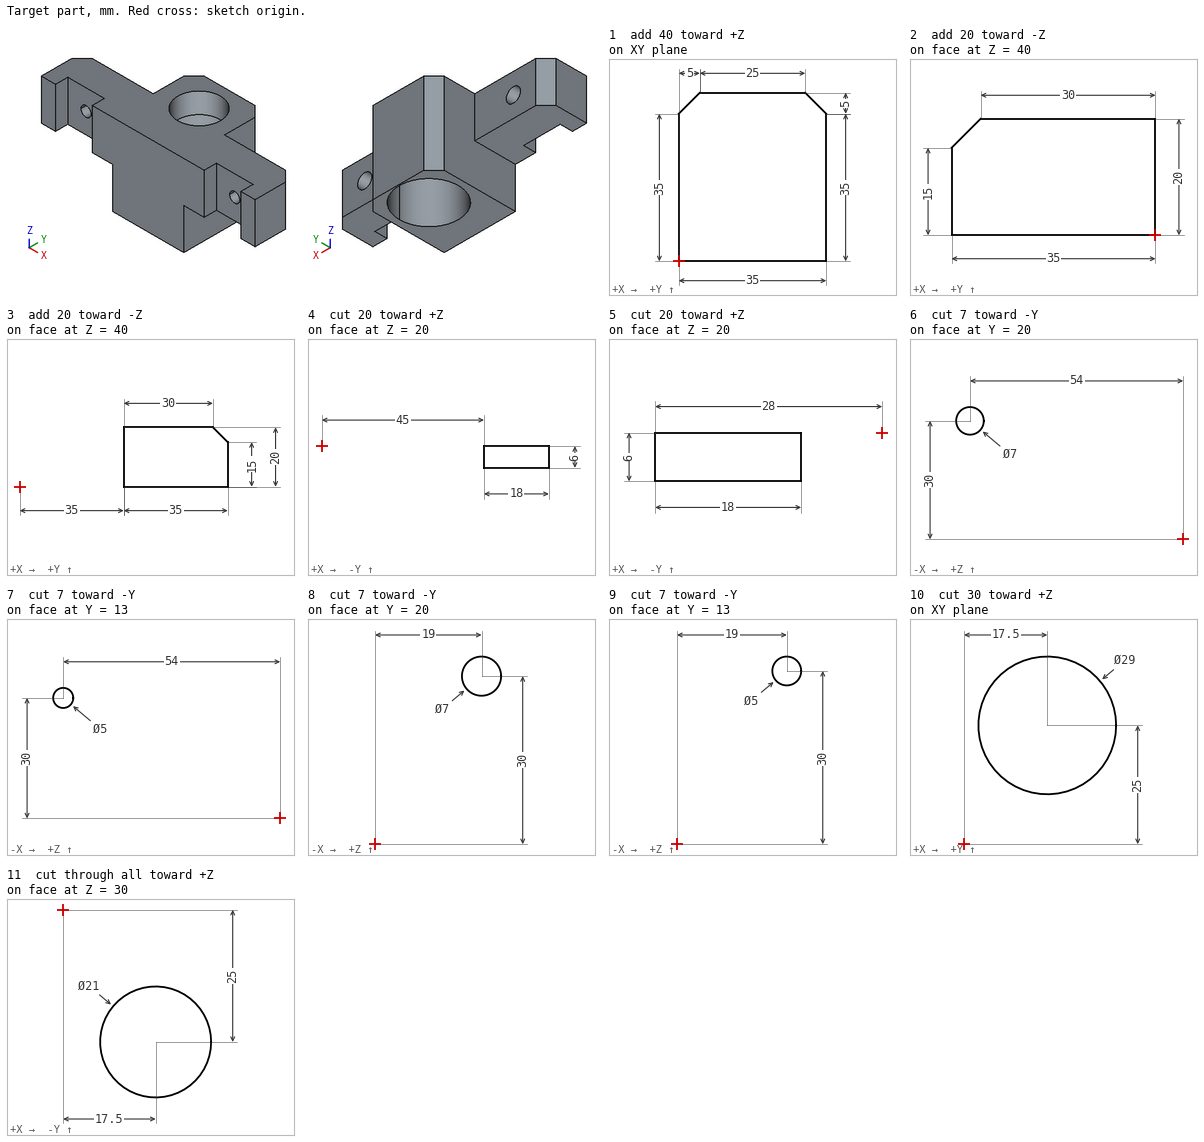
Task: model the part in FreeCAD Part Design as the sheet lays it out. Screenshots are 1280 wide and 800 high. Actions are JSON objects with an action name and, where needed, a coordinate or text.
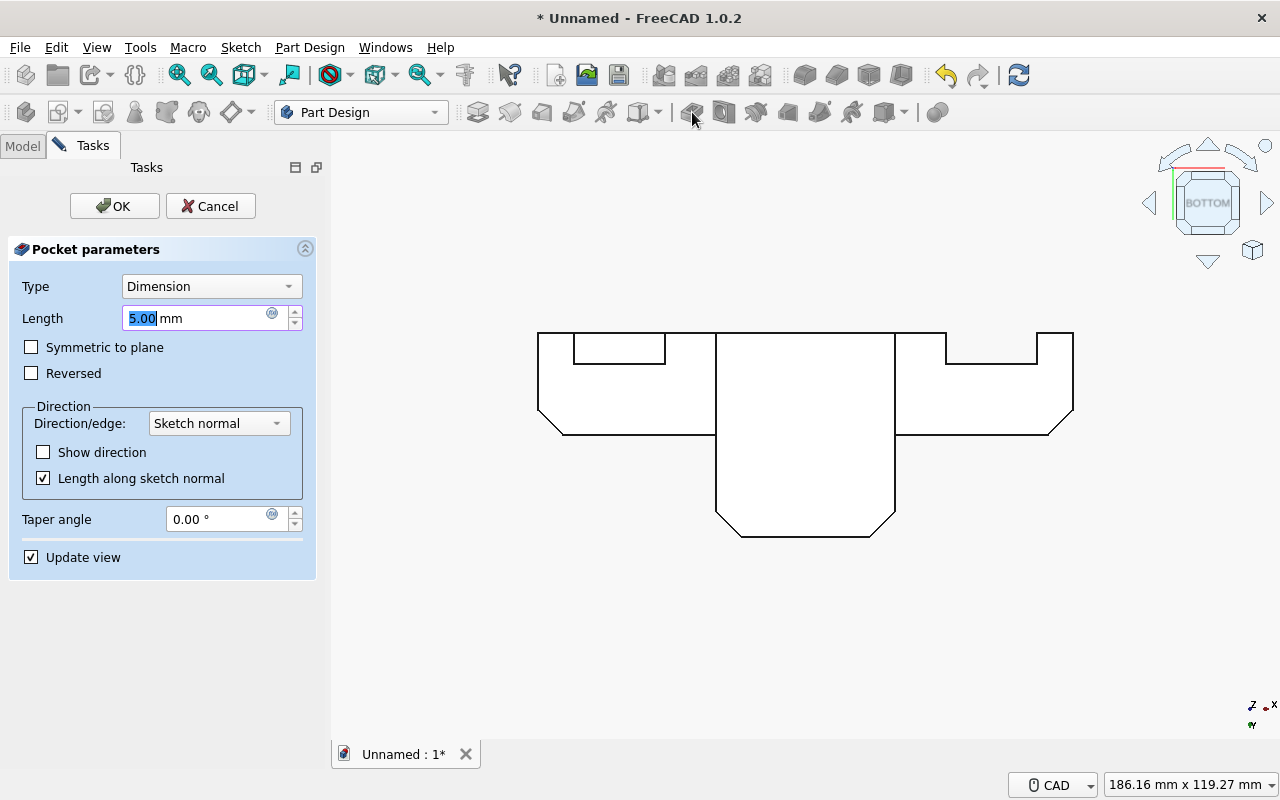
{"action": "type", "text": "20"}
{"action": "key", "text": "Tab"}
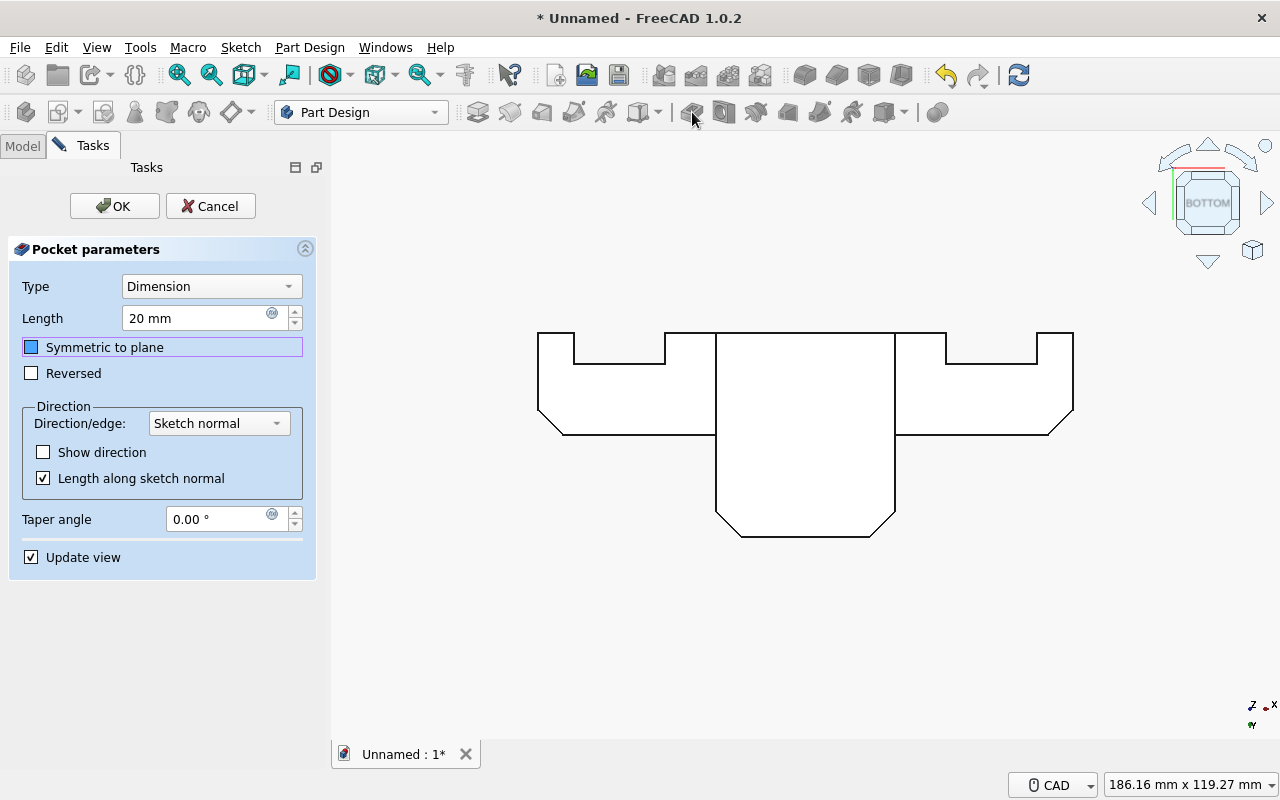
{"action": "left_click", "coordinate": [115, 206]}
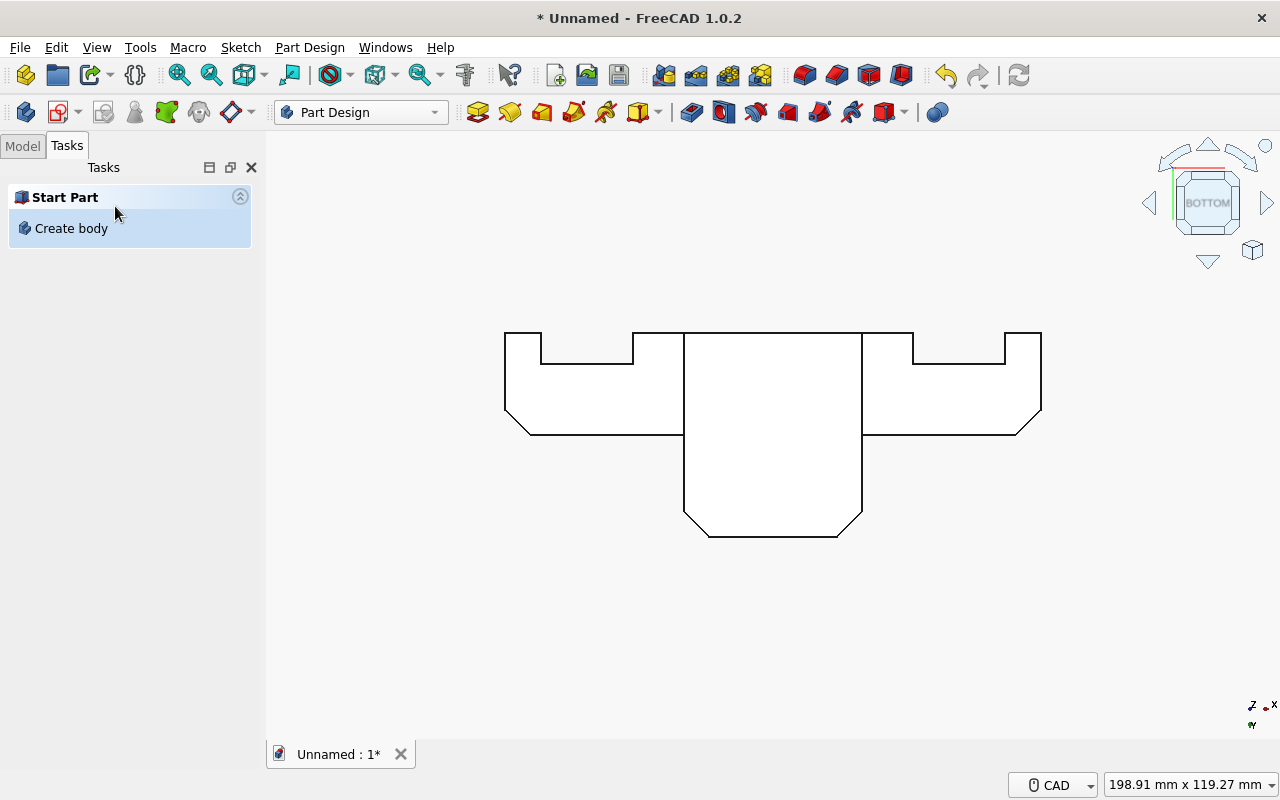
{"action": "key", "text": "4"}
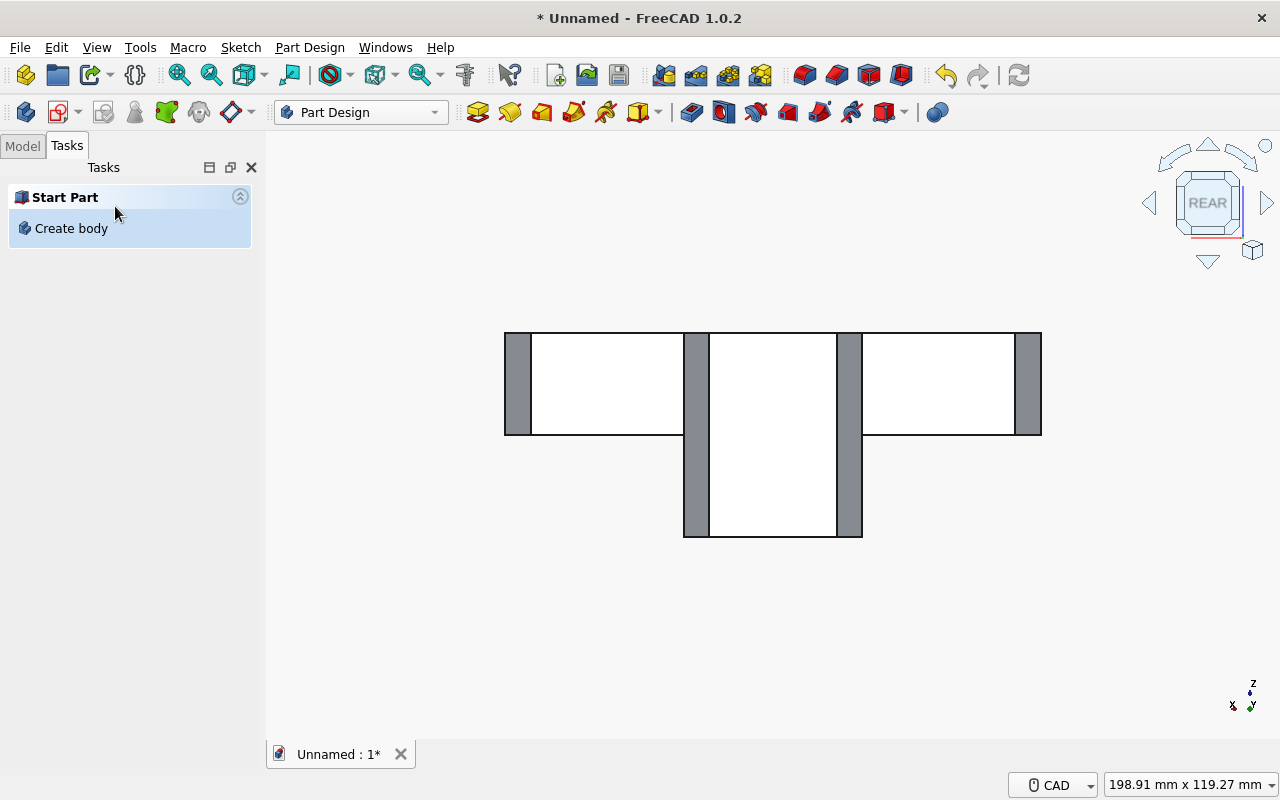
{"action": "left_click", "coordinate": [585, 383]}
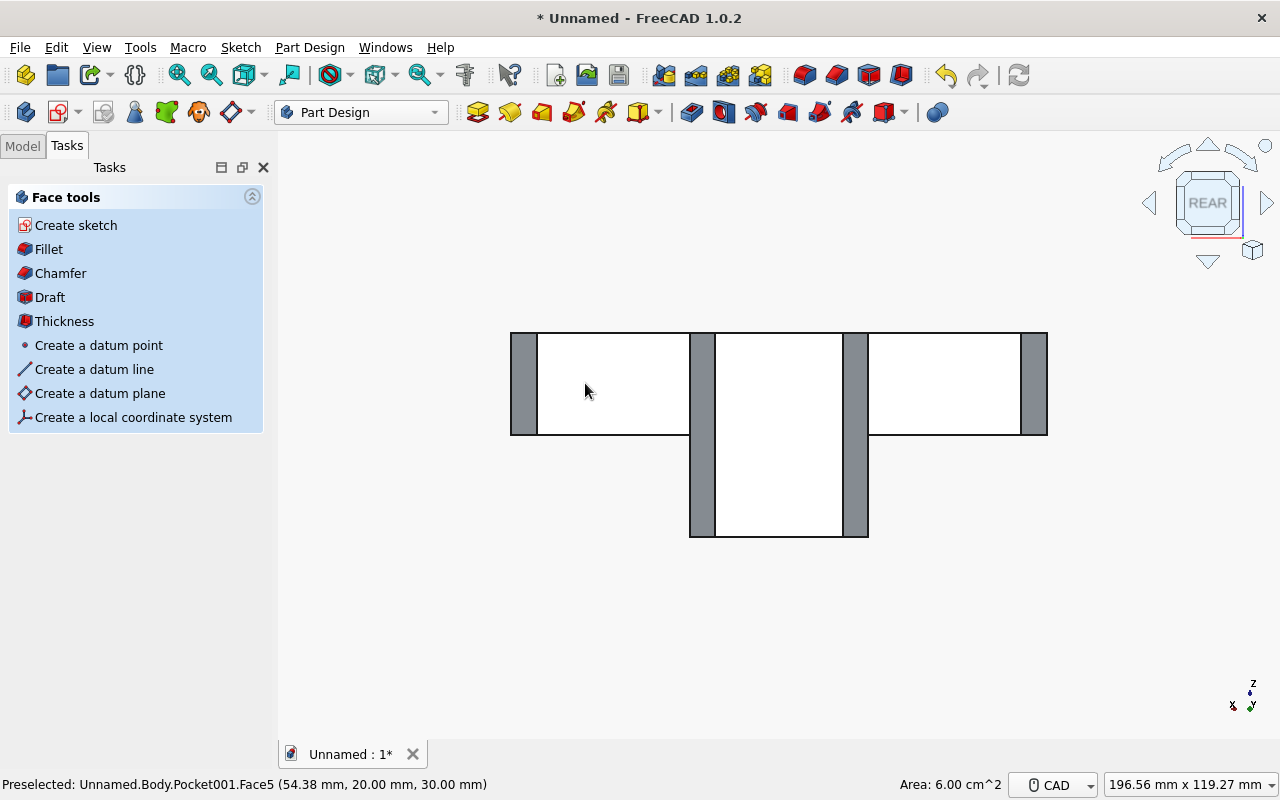
{"action": "left_click", "coordinate": [58, 112]}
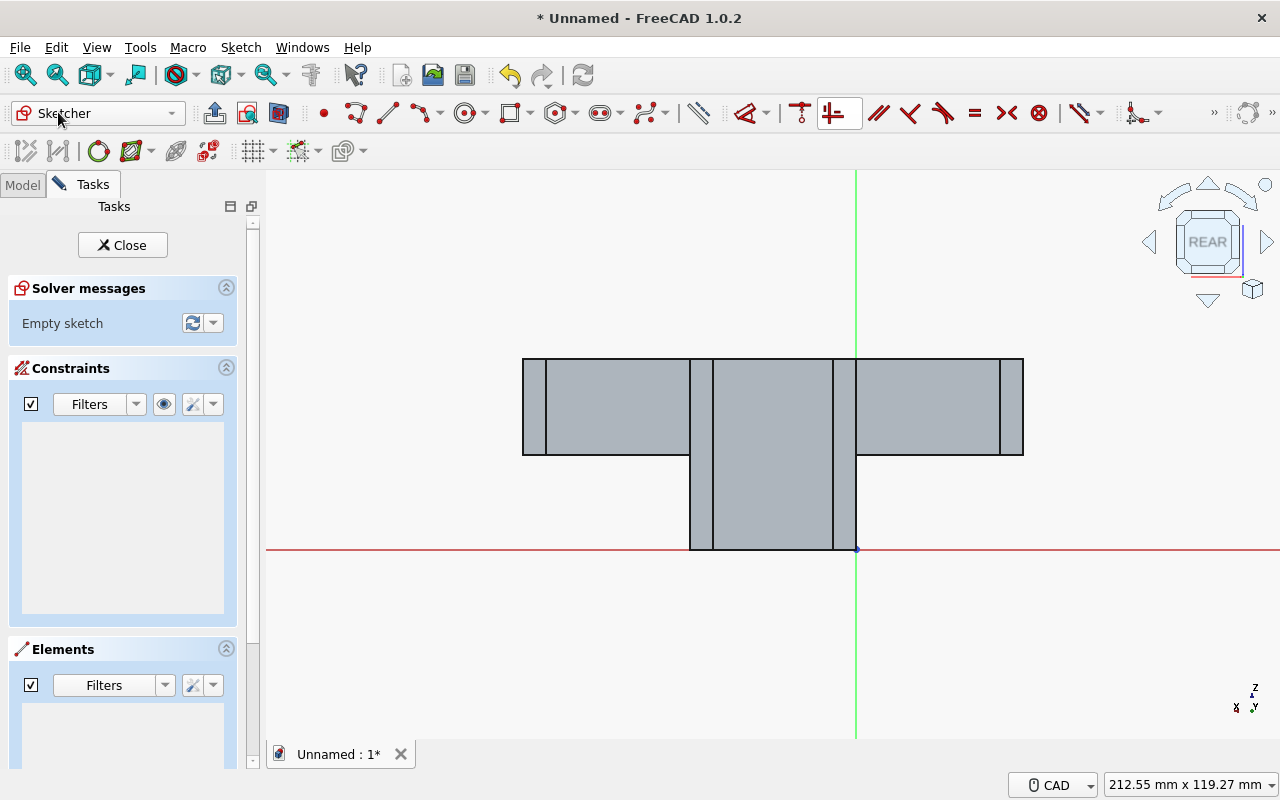
{"action": "scroll", "coordinate": [588, 402], "scroll_direction": "up", "scroll_amount": 12}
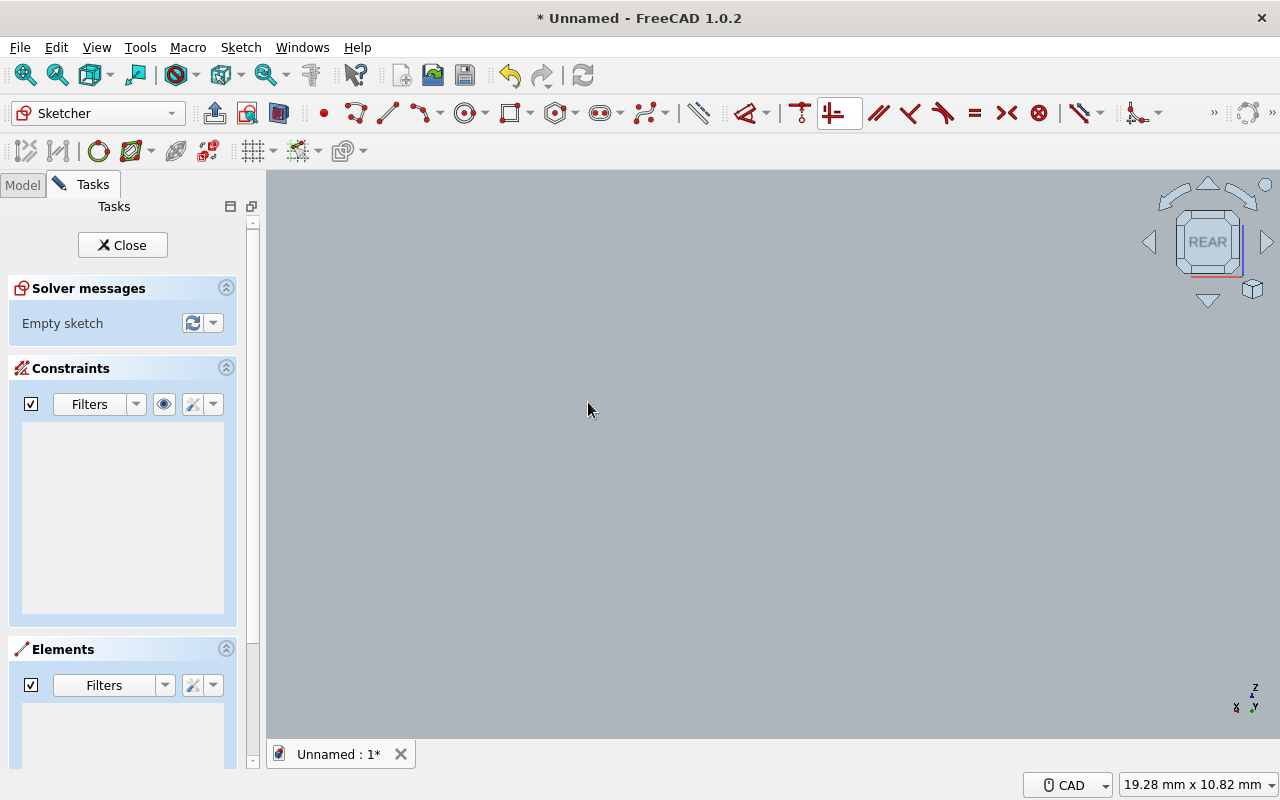
{"action": "left_click", "coordinate": [466, 114]}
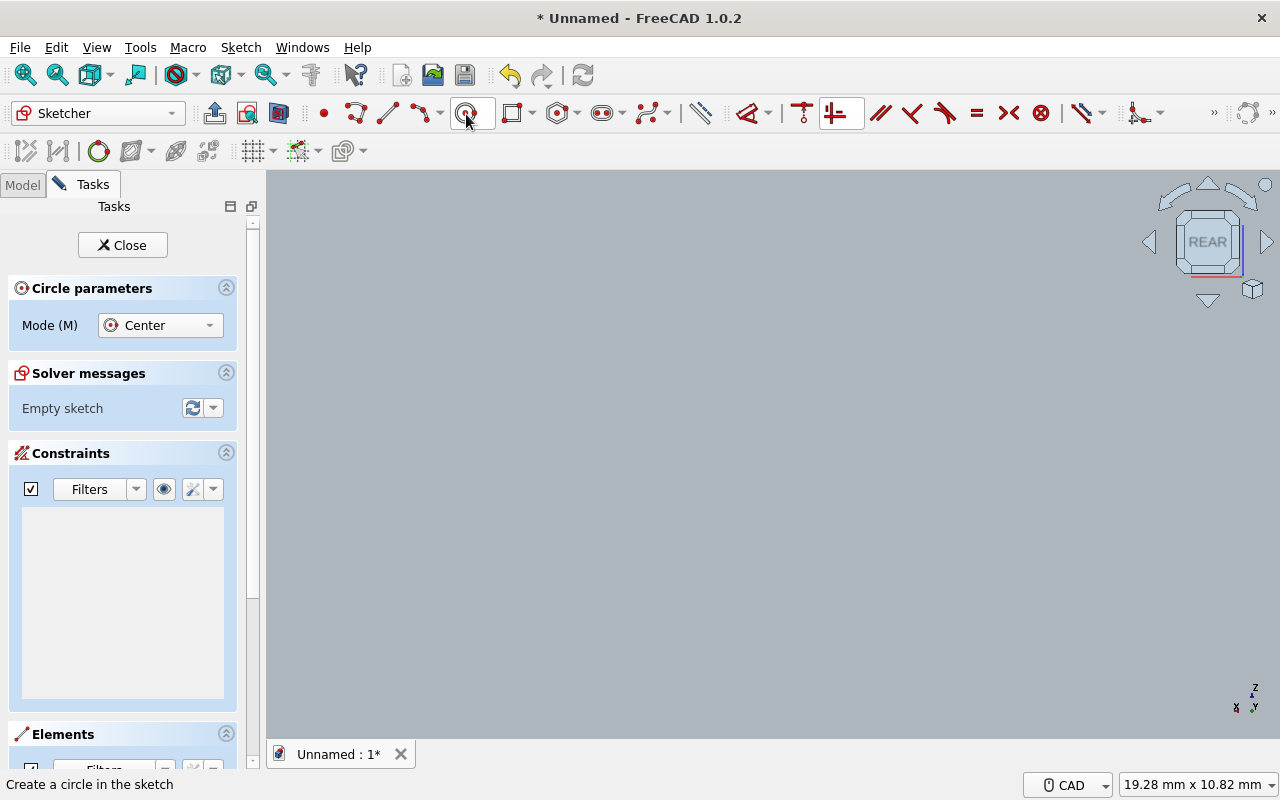
{"action": "left_click", "coordinate": [705, 451]}
{"action": "left_click", "coordinate": [835, 321]}
{"action": "key", "text": "Escape"}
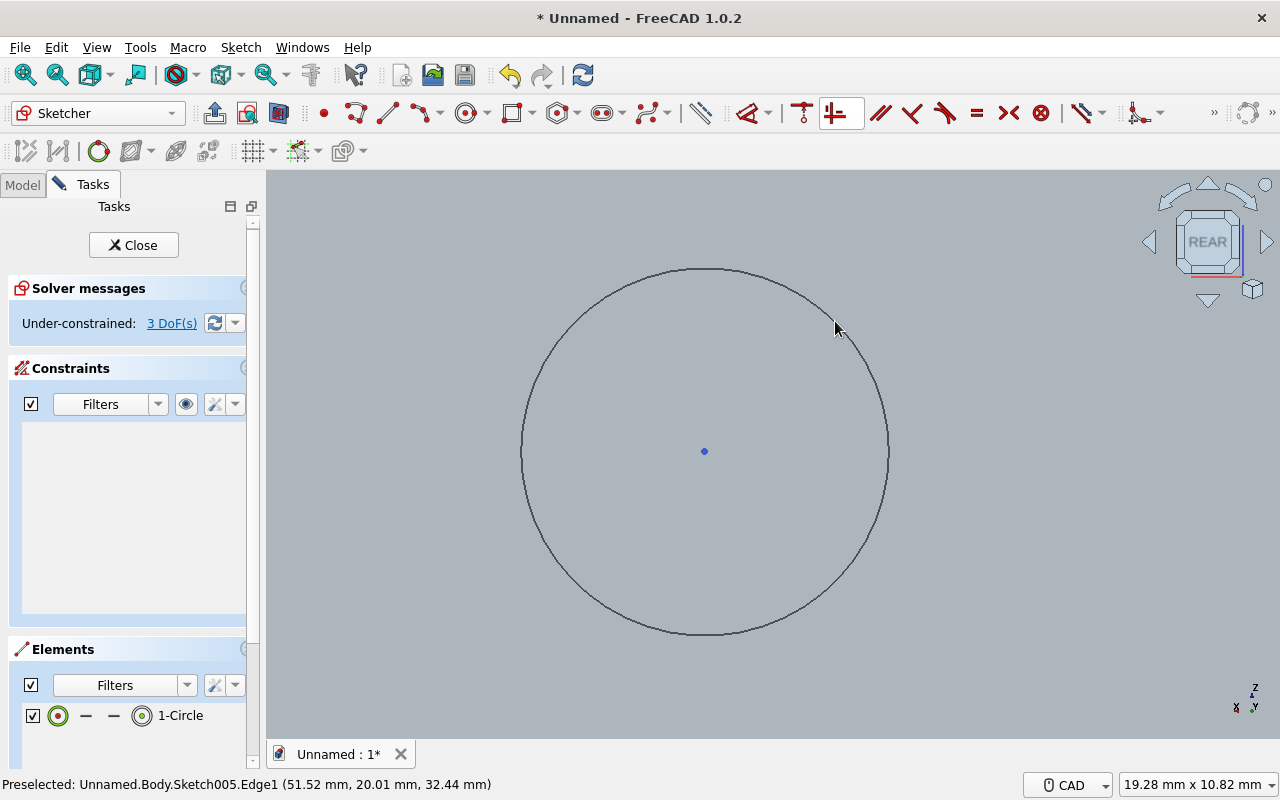
{"action": "left_click", "coordinate": [748, 114]}